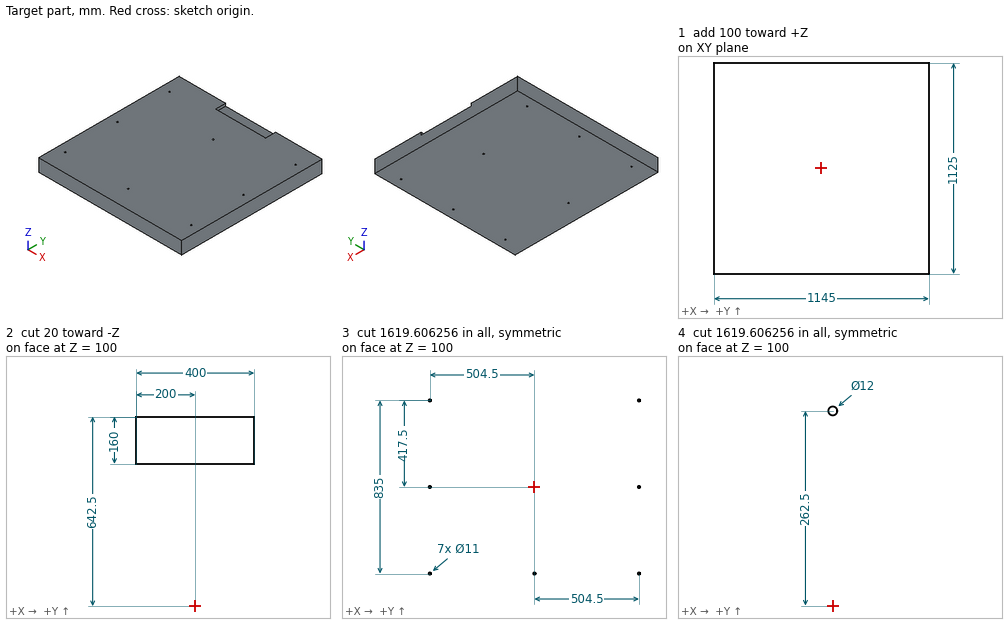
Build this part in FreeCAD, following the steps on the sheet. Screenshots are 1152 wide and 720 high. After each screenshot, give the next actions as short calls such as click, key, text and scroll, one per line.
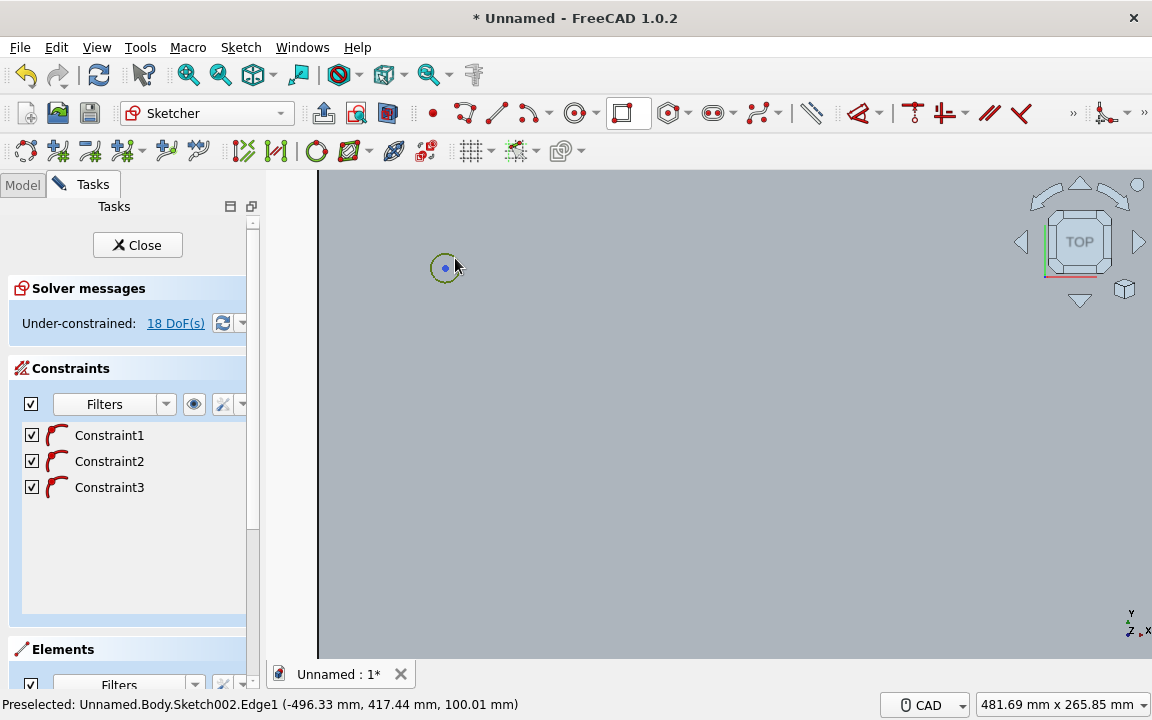
scroll(456, 259, down, 8)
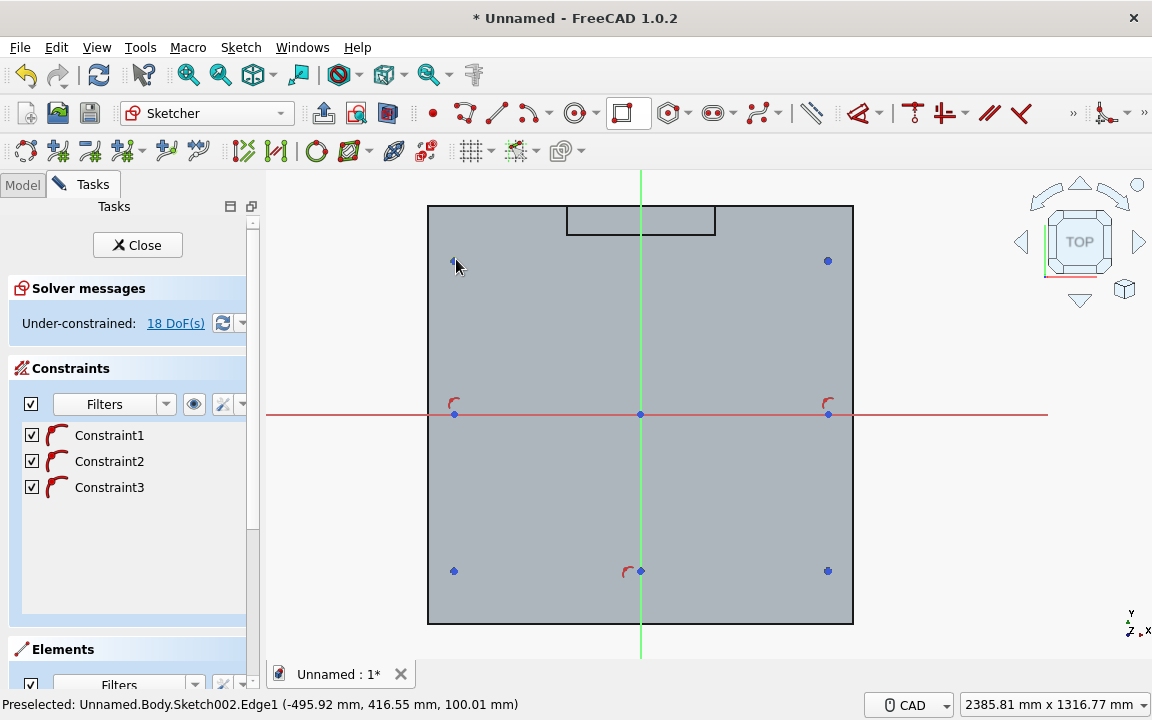
scroll(456, 569, up, 8)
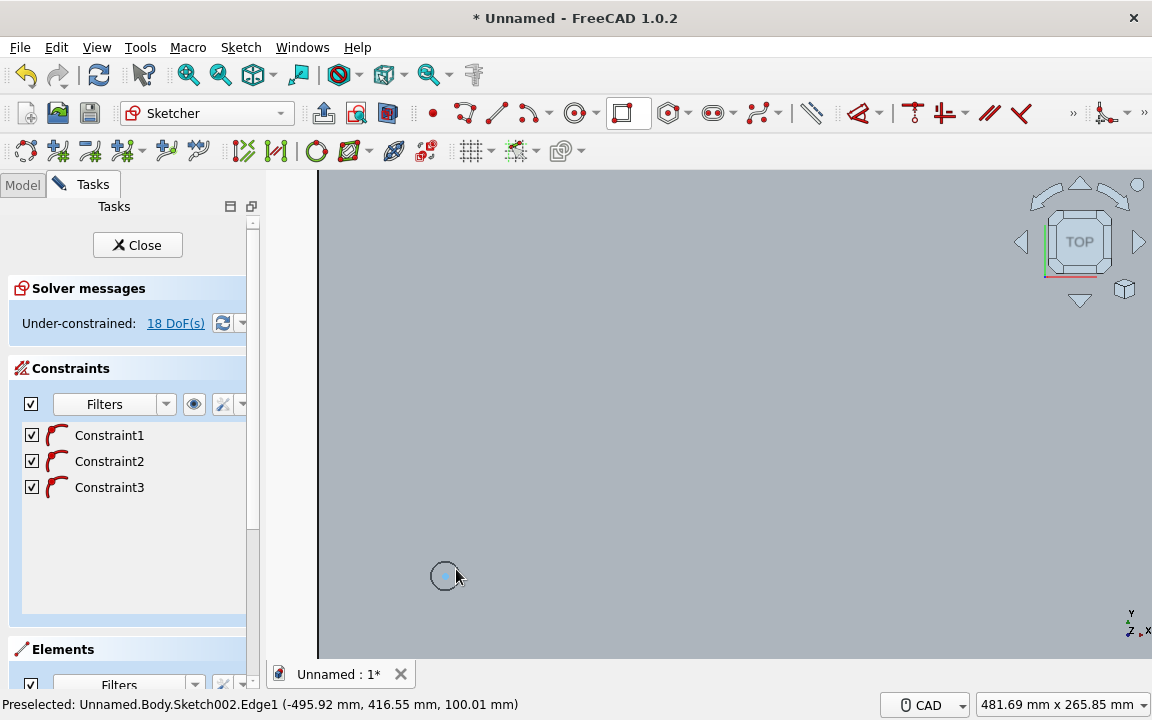
click(455, 566)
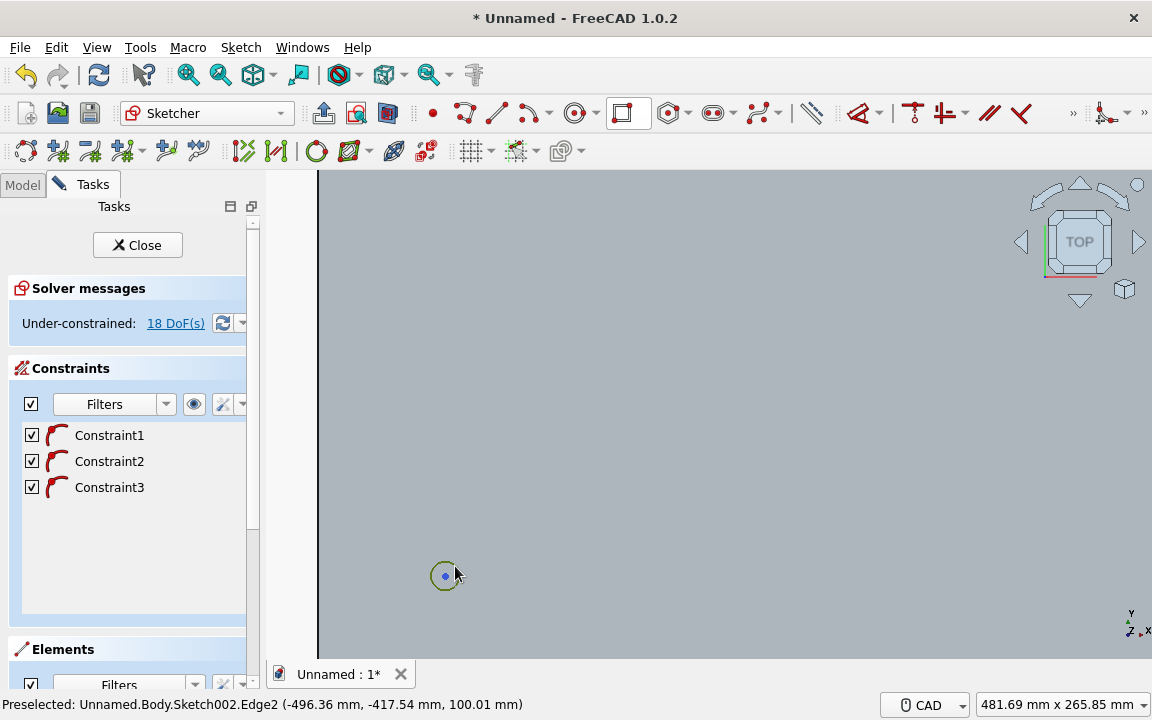
scroll(456, 570, down, 8)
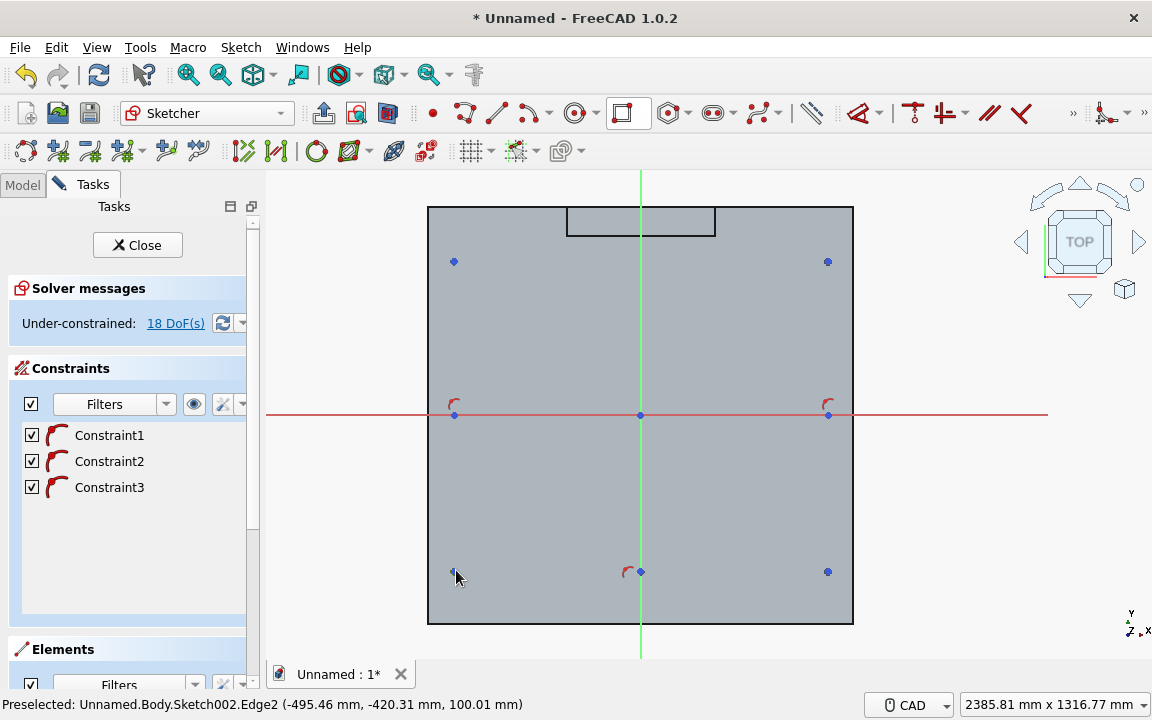
scroll(830, 570, up, 8)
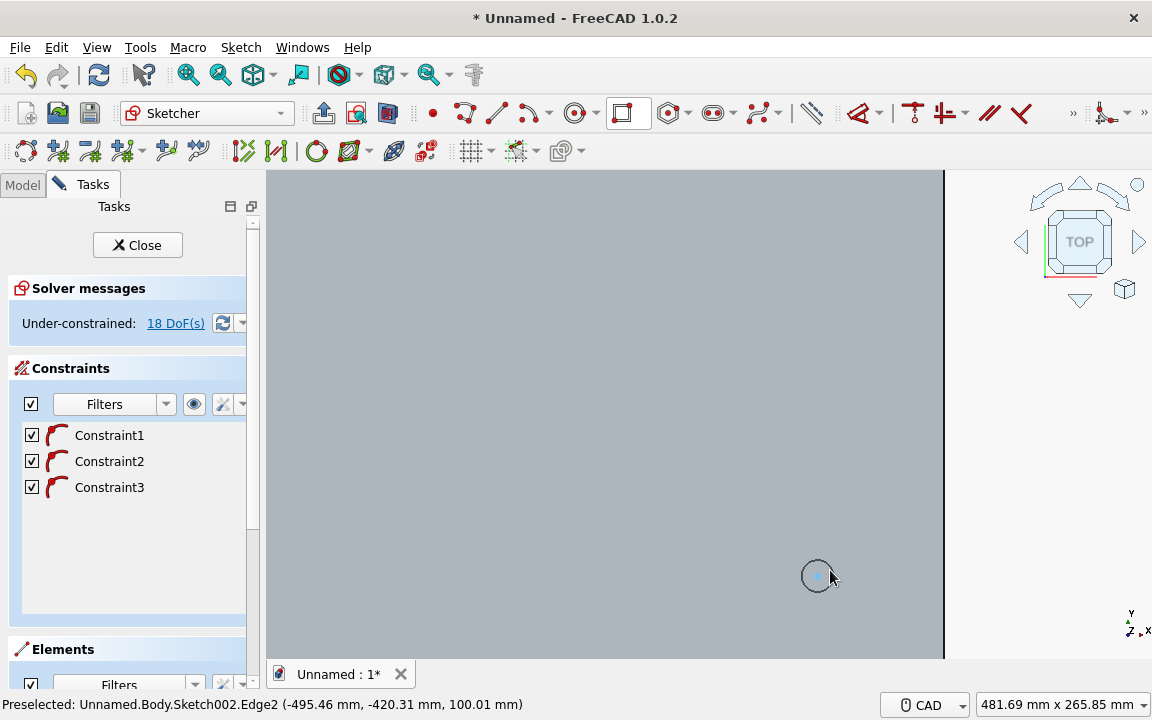
click(829, 565)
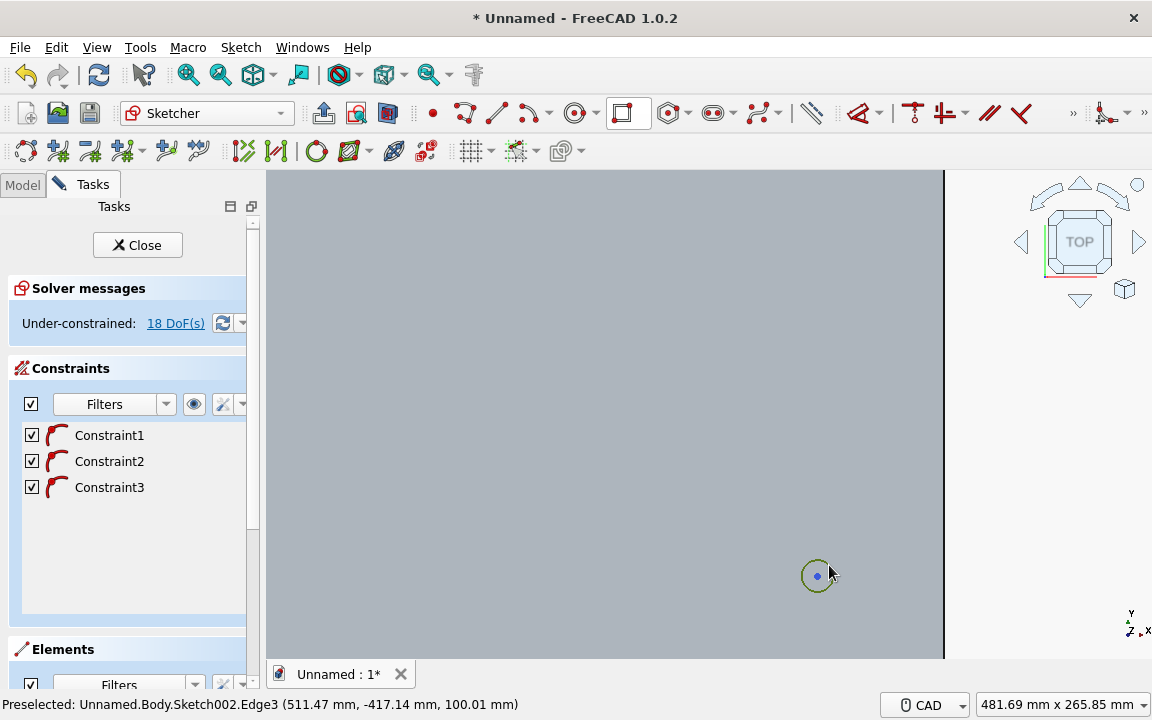
scroll(830, 570, down, 8)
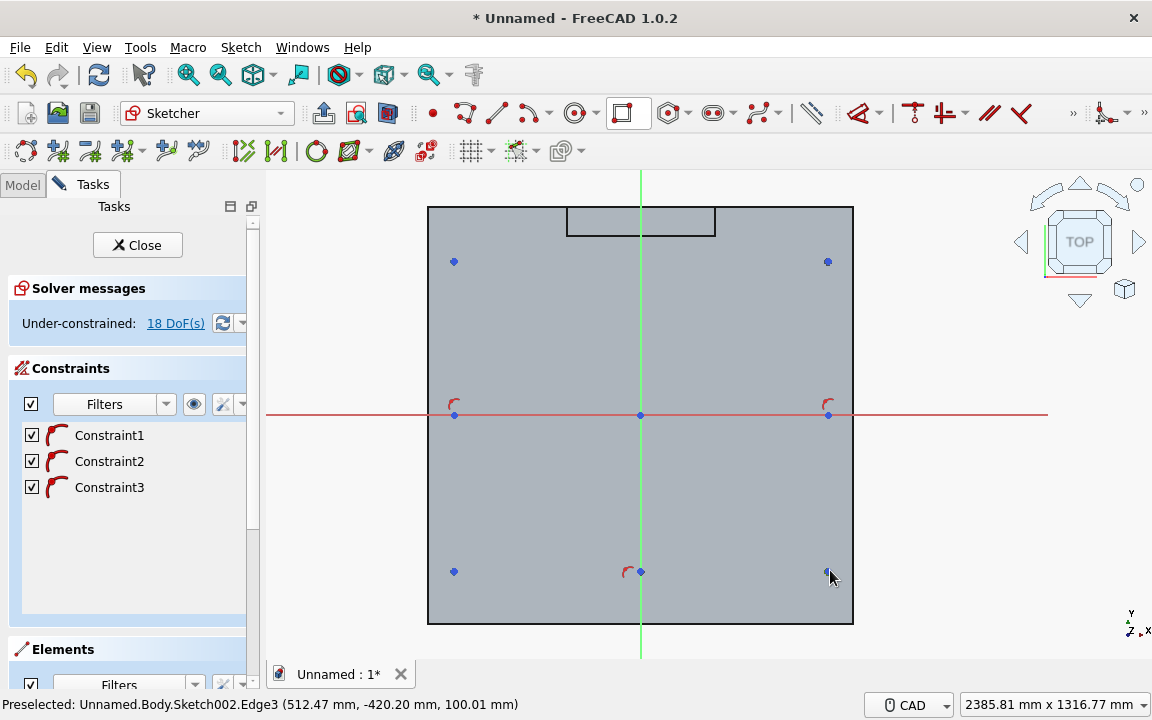
scroll(830, 260, up, 8)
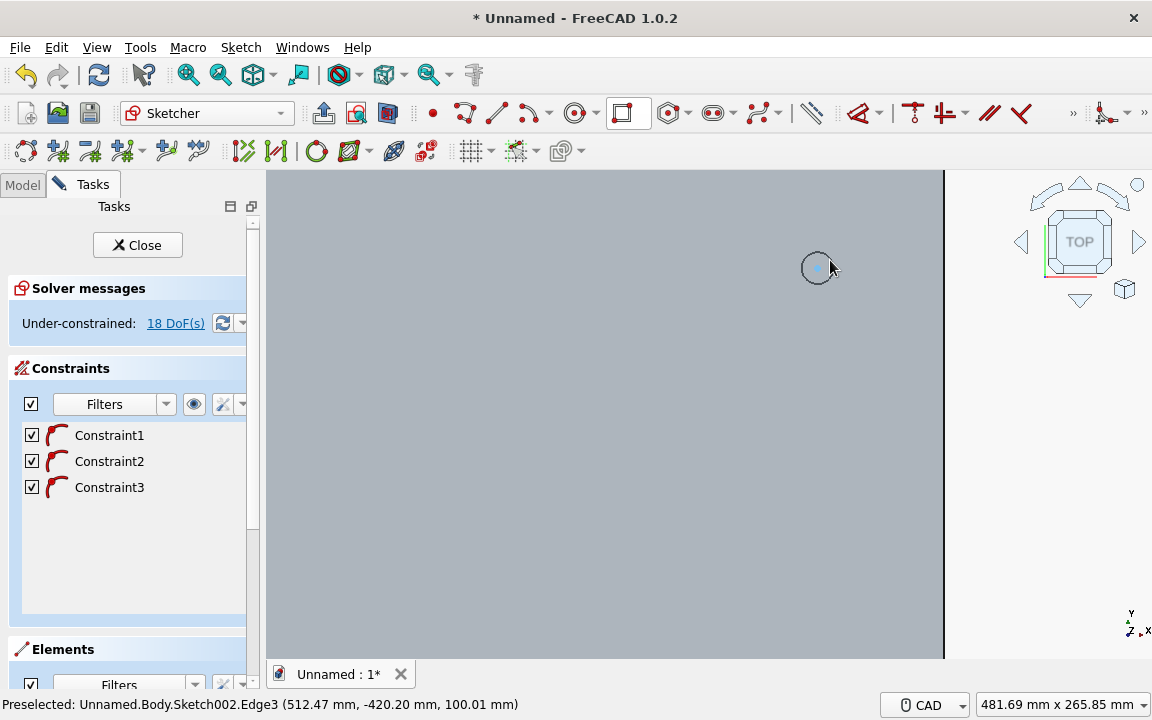
click(829, 257)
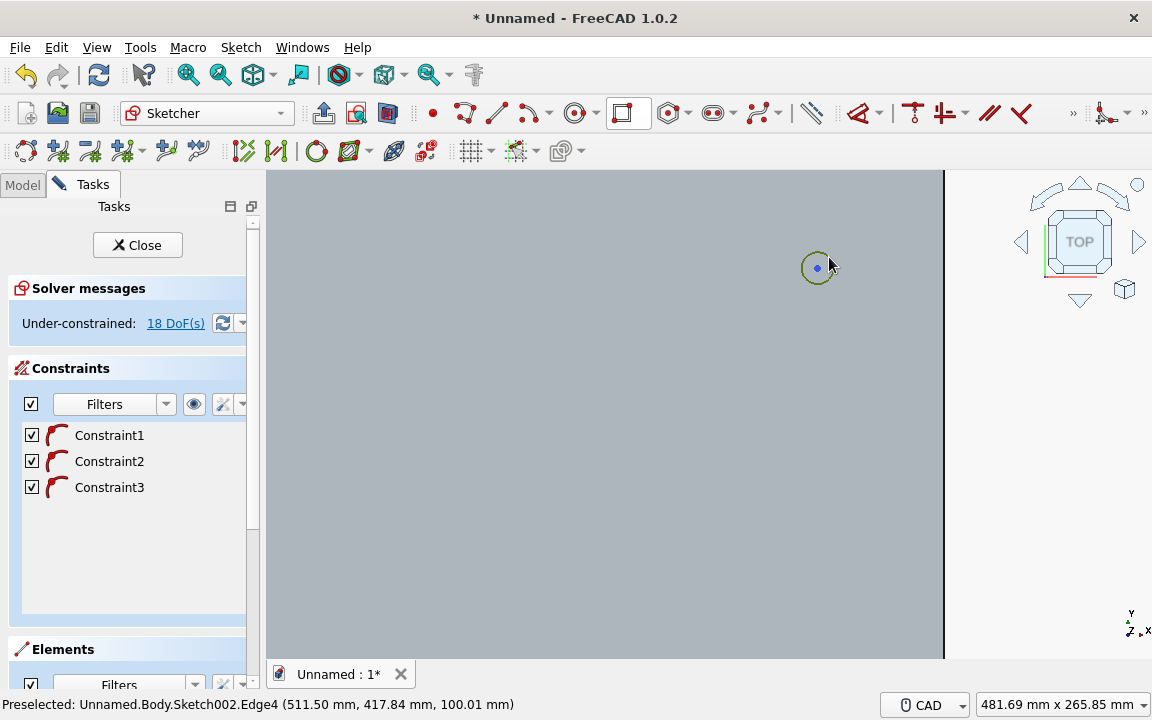
scroll(830, 259, down, 8)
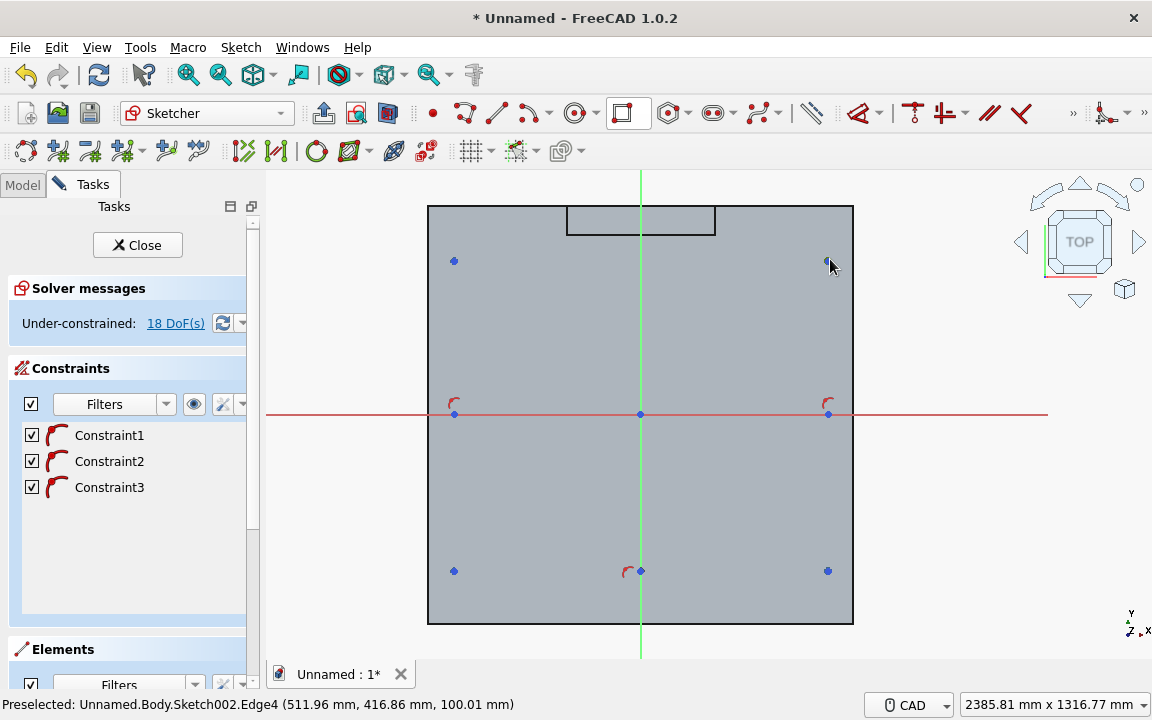
scroll(643, 569, up, 10)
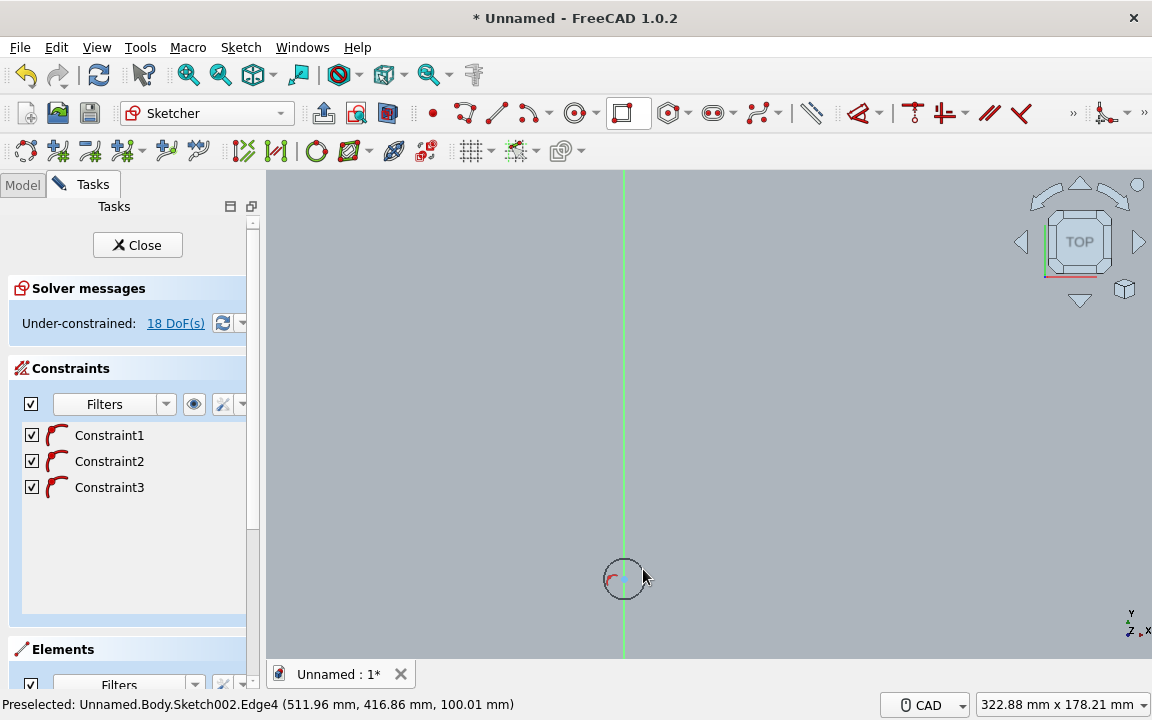
click(639, 565)